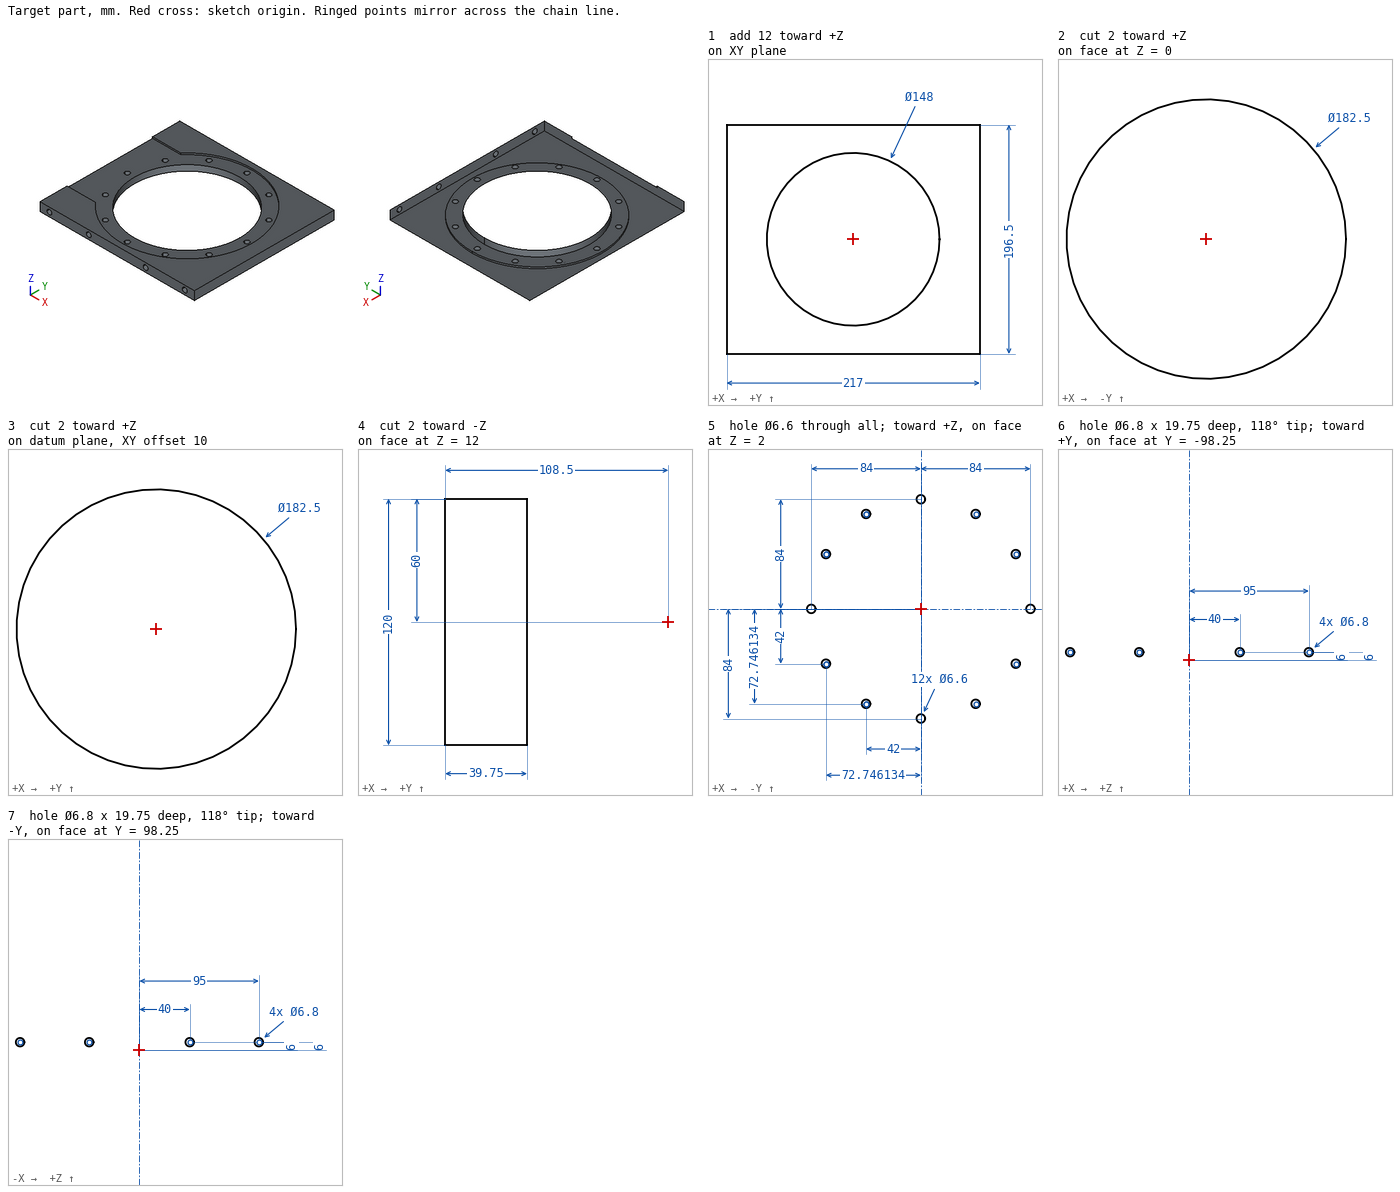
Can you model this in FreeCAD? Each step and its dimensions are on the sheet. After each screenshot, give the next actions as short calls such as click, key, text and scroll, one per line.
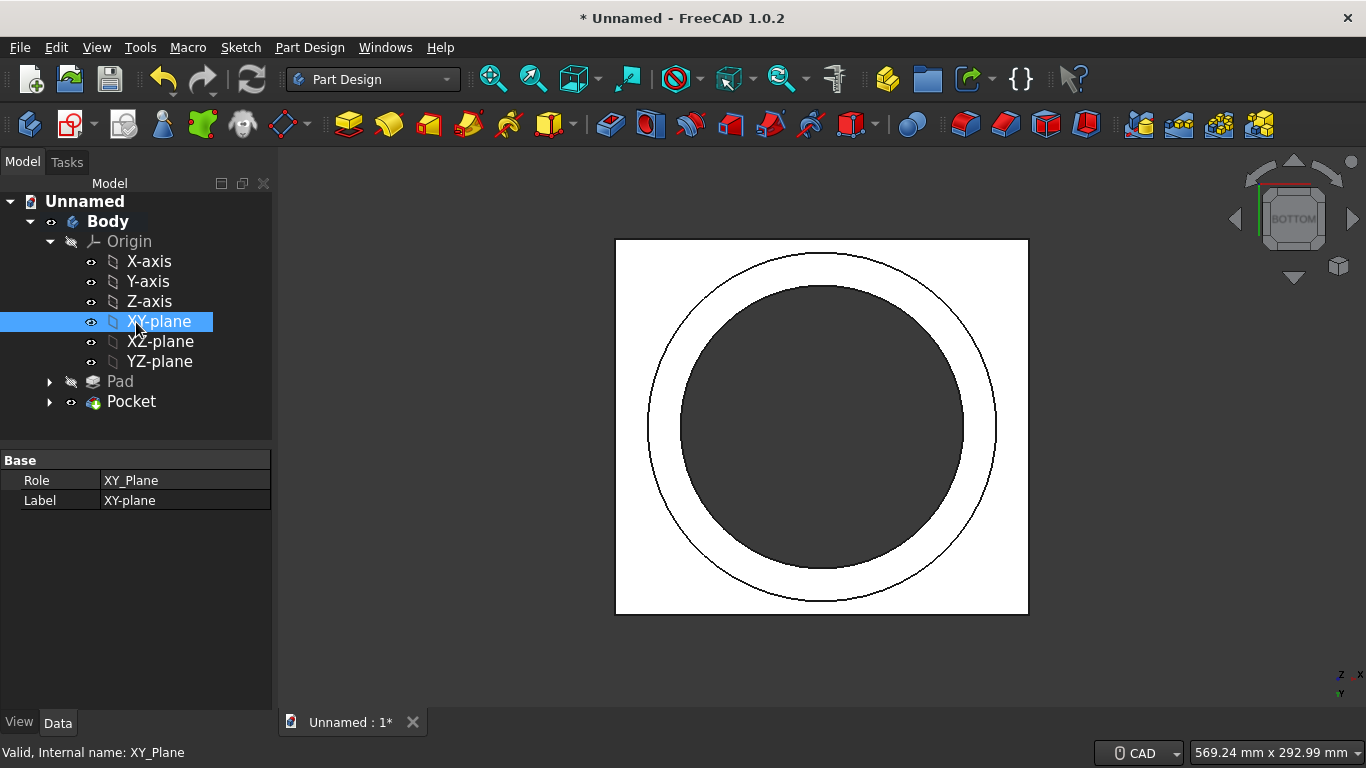
click(284, 124)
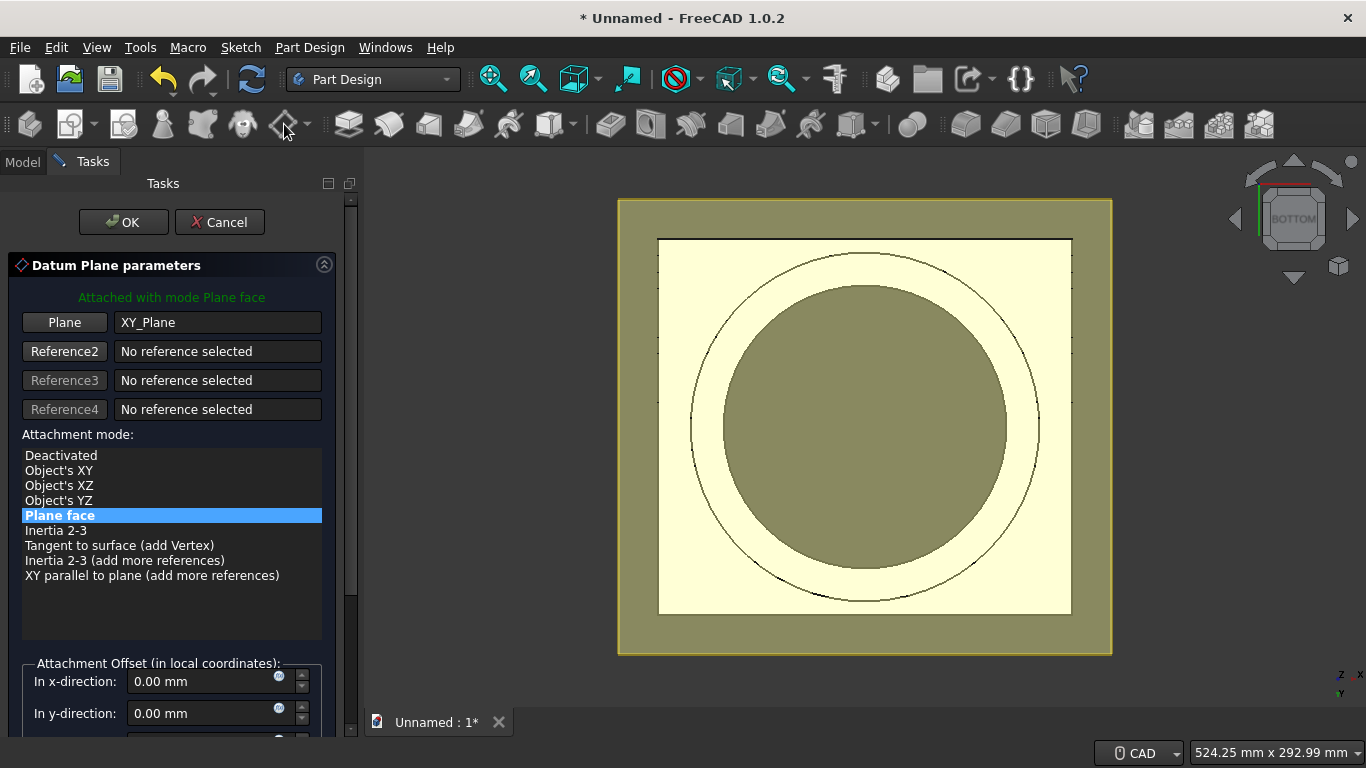
scroll(351, 464, down, 2)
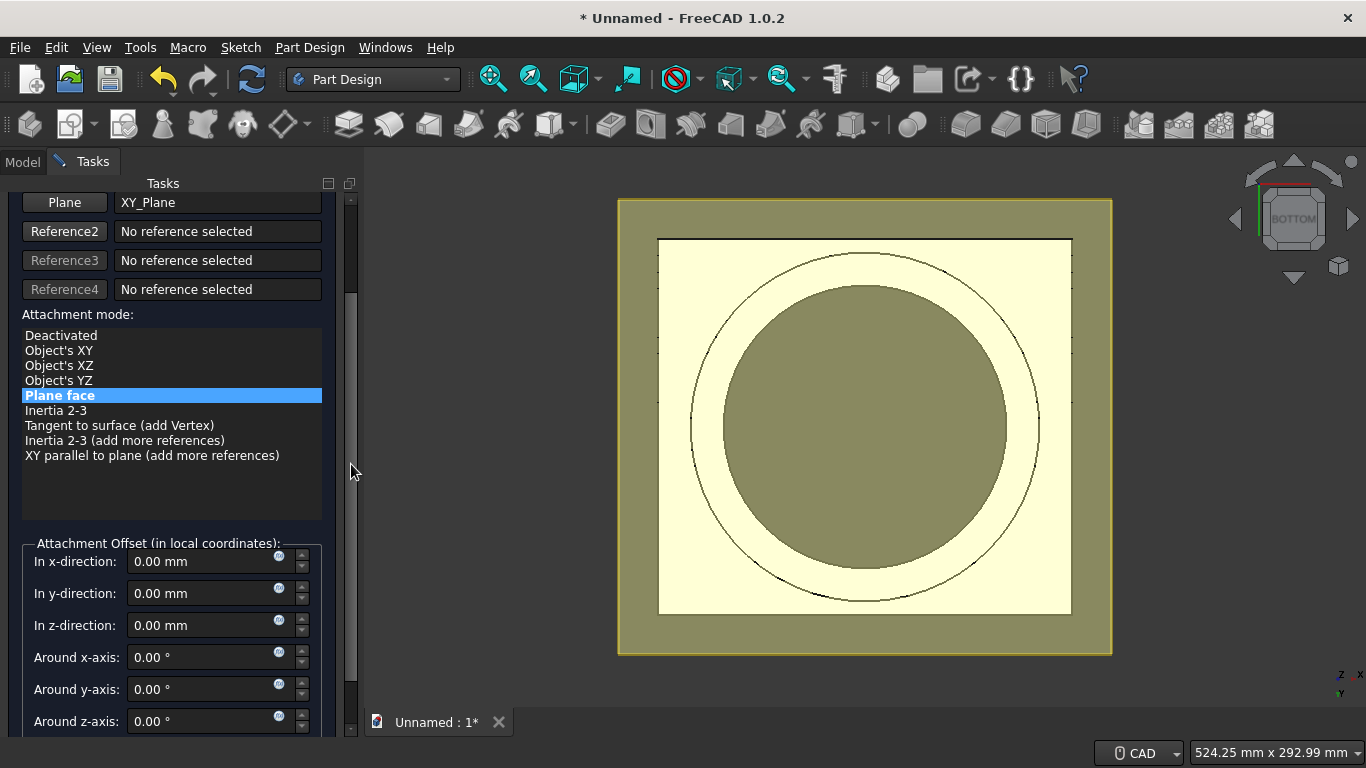
triple_click(210, 625)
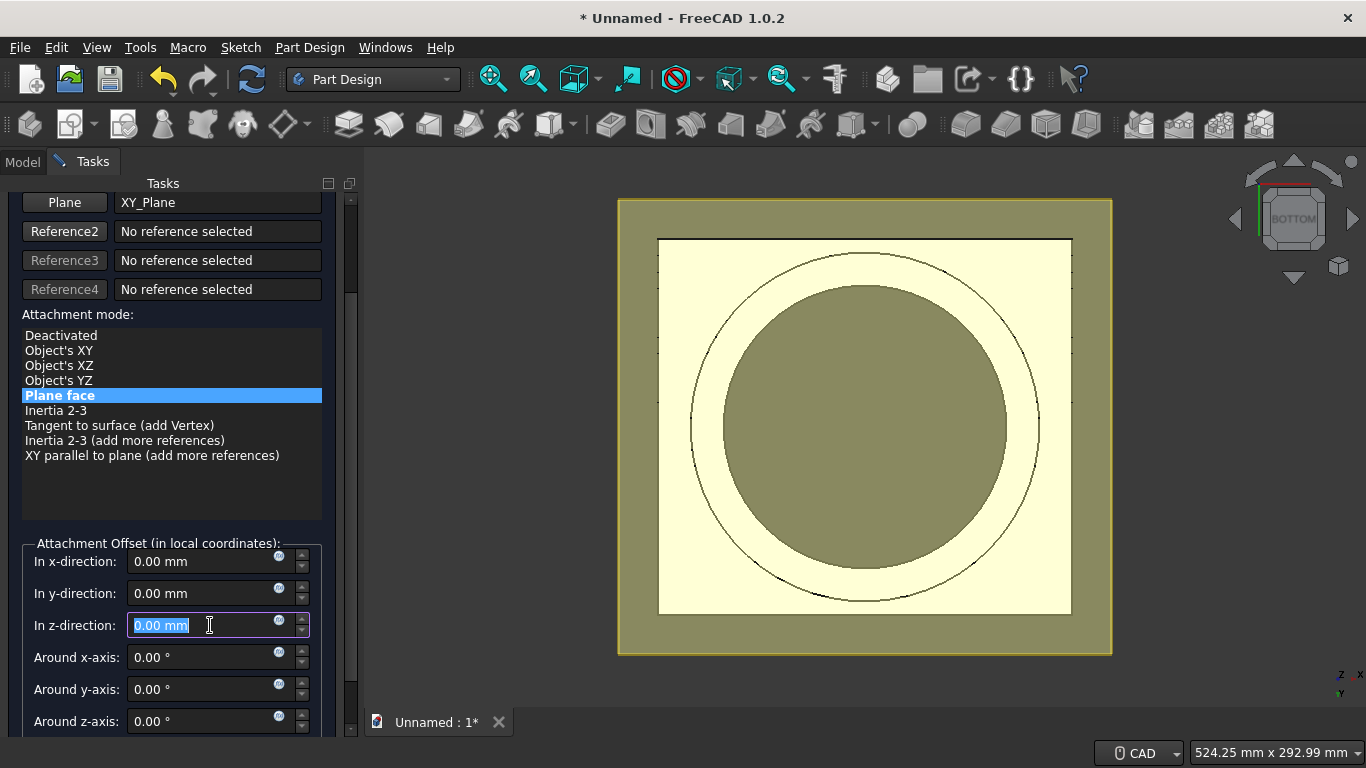
text(10)
key(Tab)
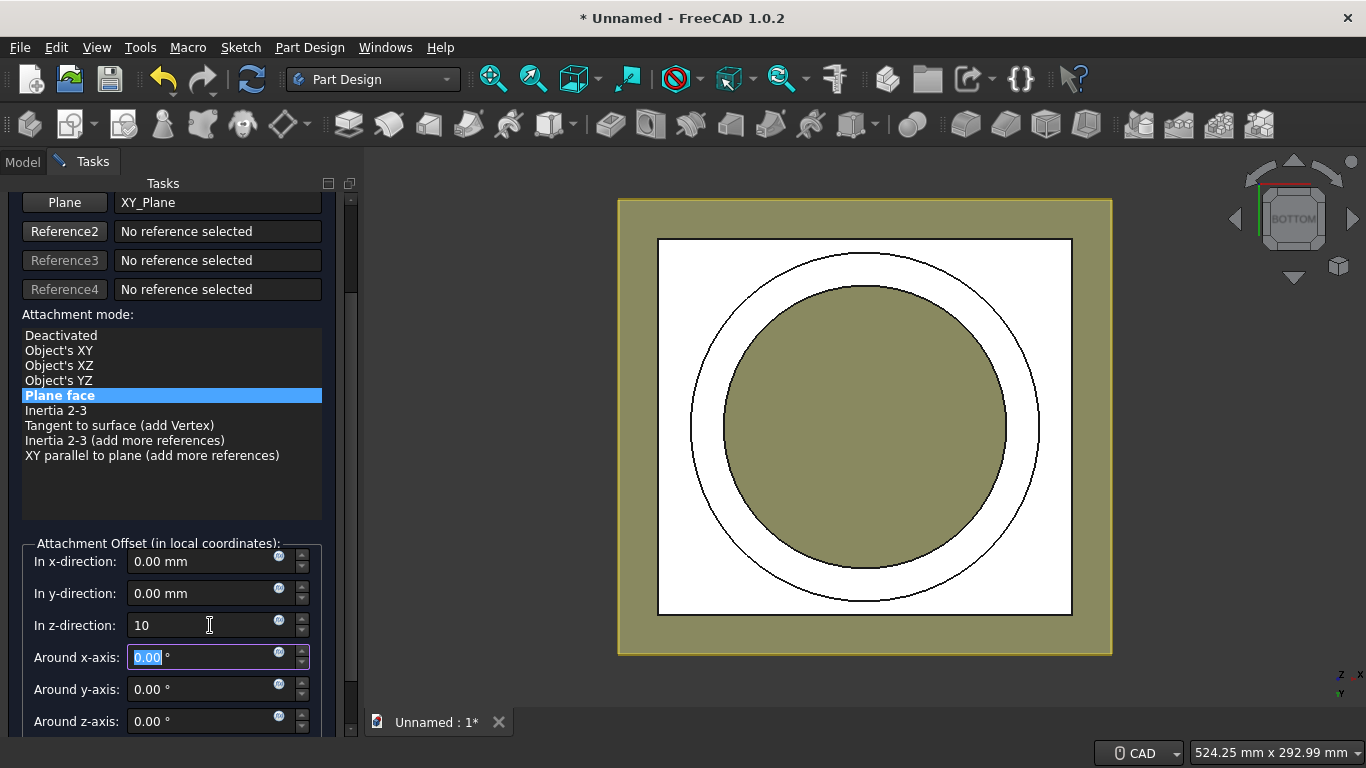
scroll(351, 464, up, 3)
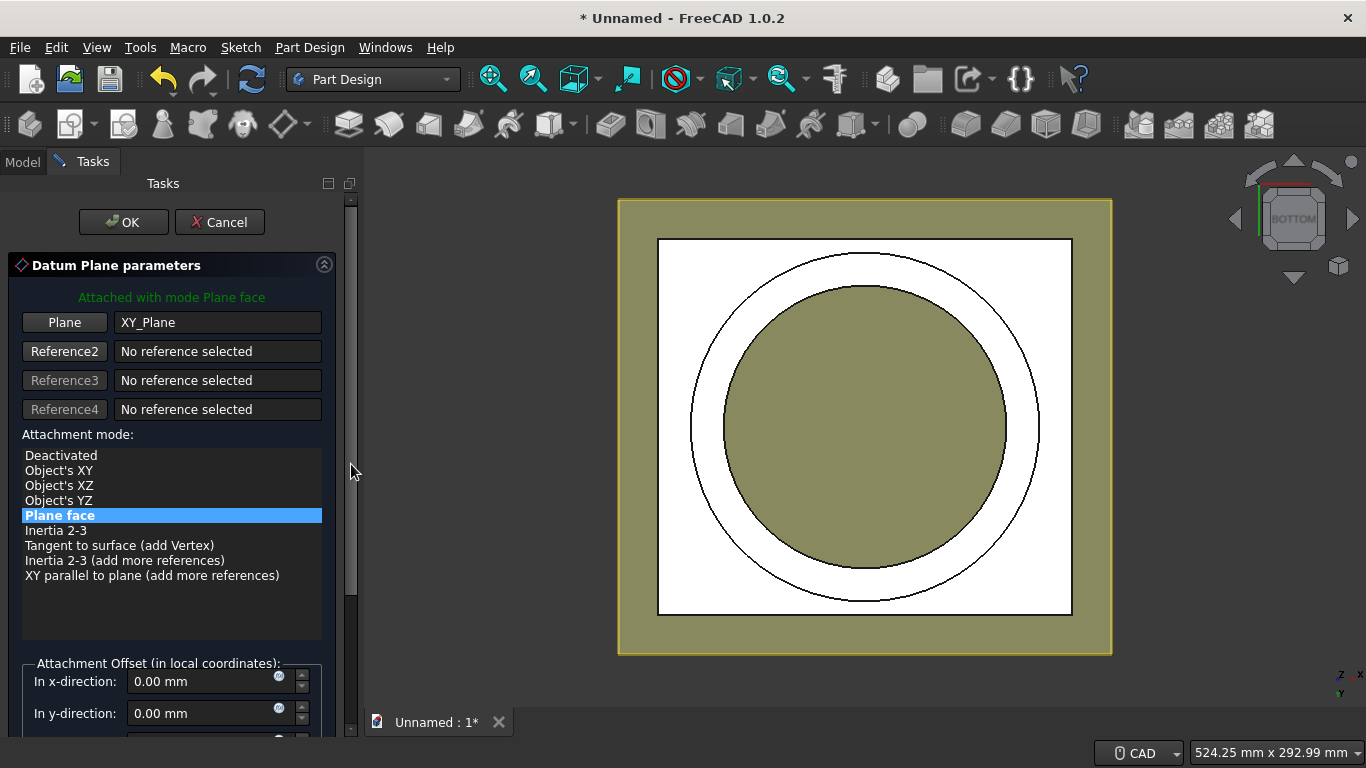
click(124, 222)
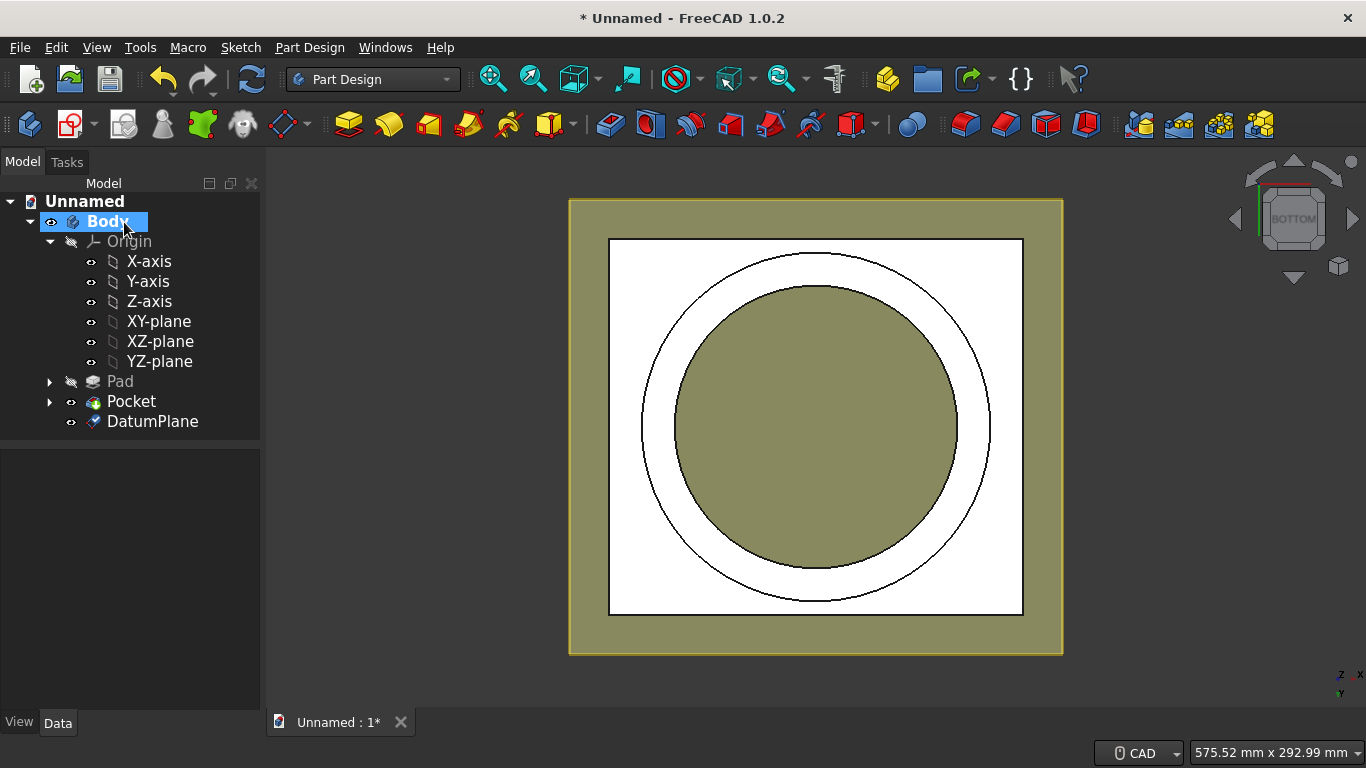
click(116, 422)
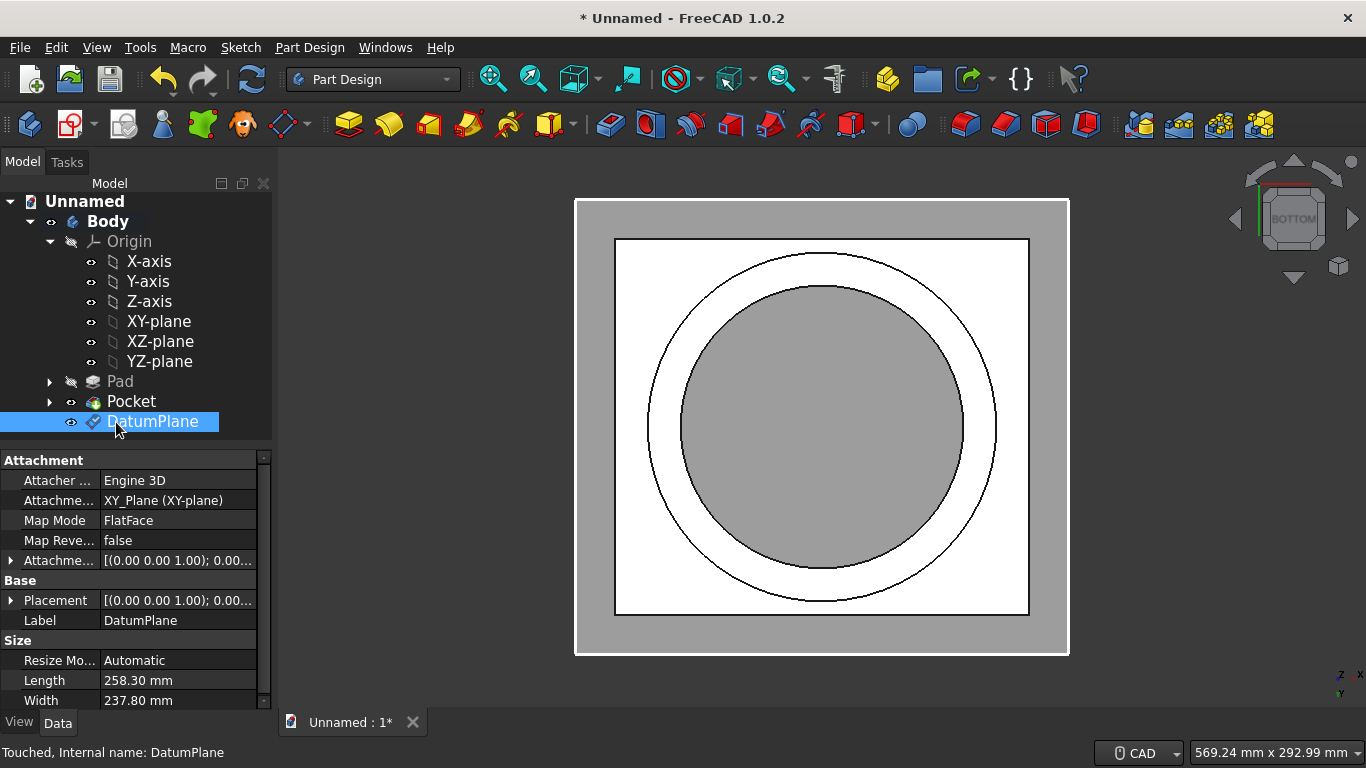
click(70, 124)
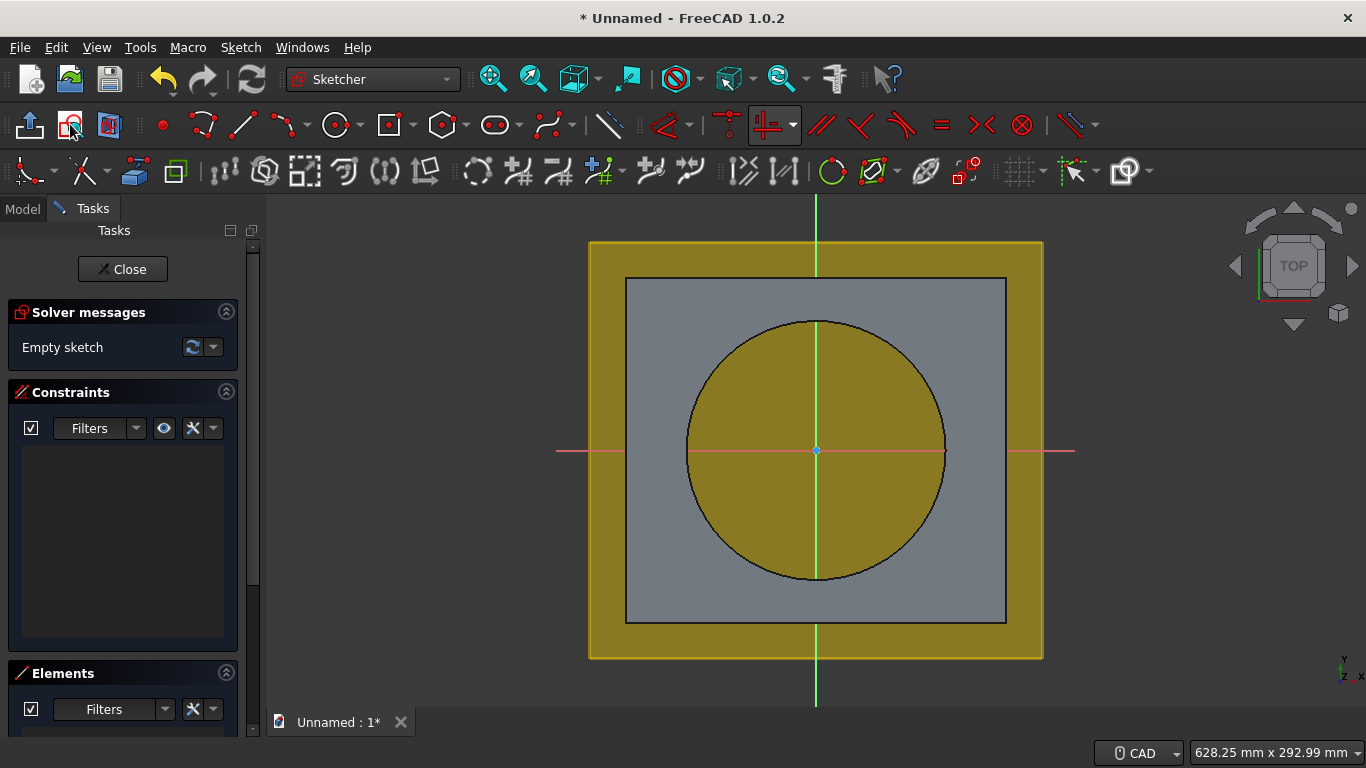
click(110, 126)